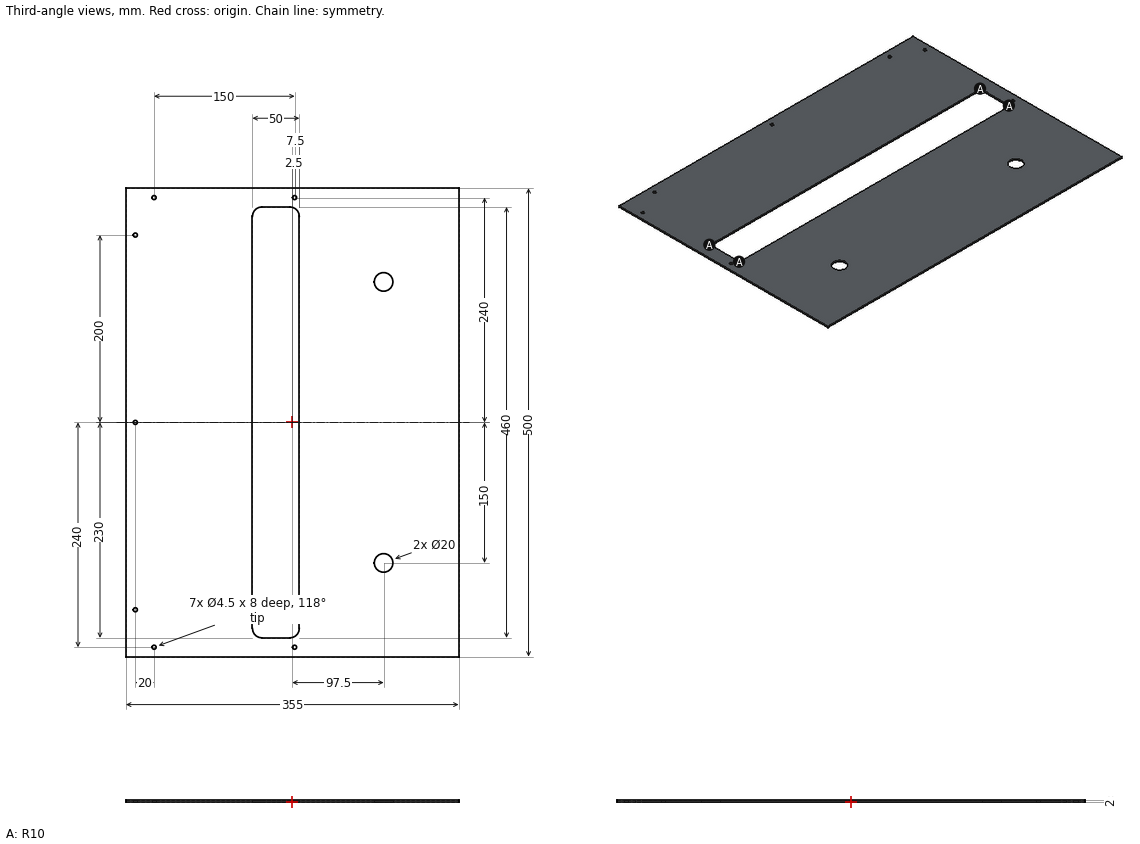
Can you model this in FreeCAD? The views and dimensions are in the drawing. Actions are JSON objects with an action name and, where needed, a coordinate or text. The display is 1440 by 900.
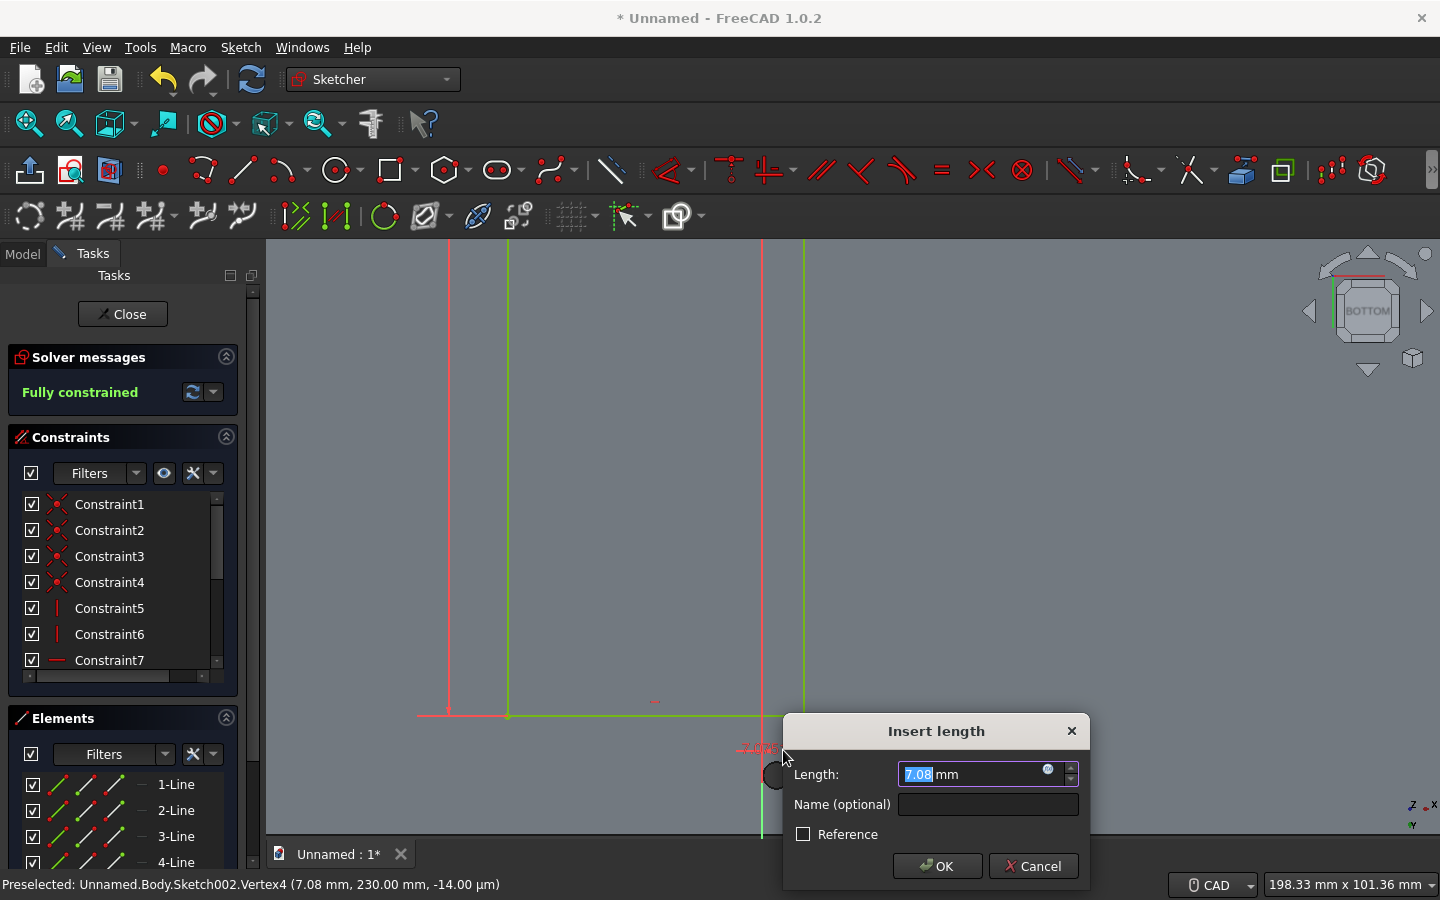
{"action": "type", "text": "7.5"}
{"action": "key", "text": "Return"}
{"action": "key", "text": "Escape"}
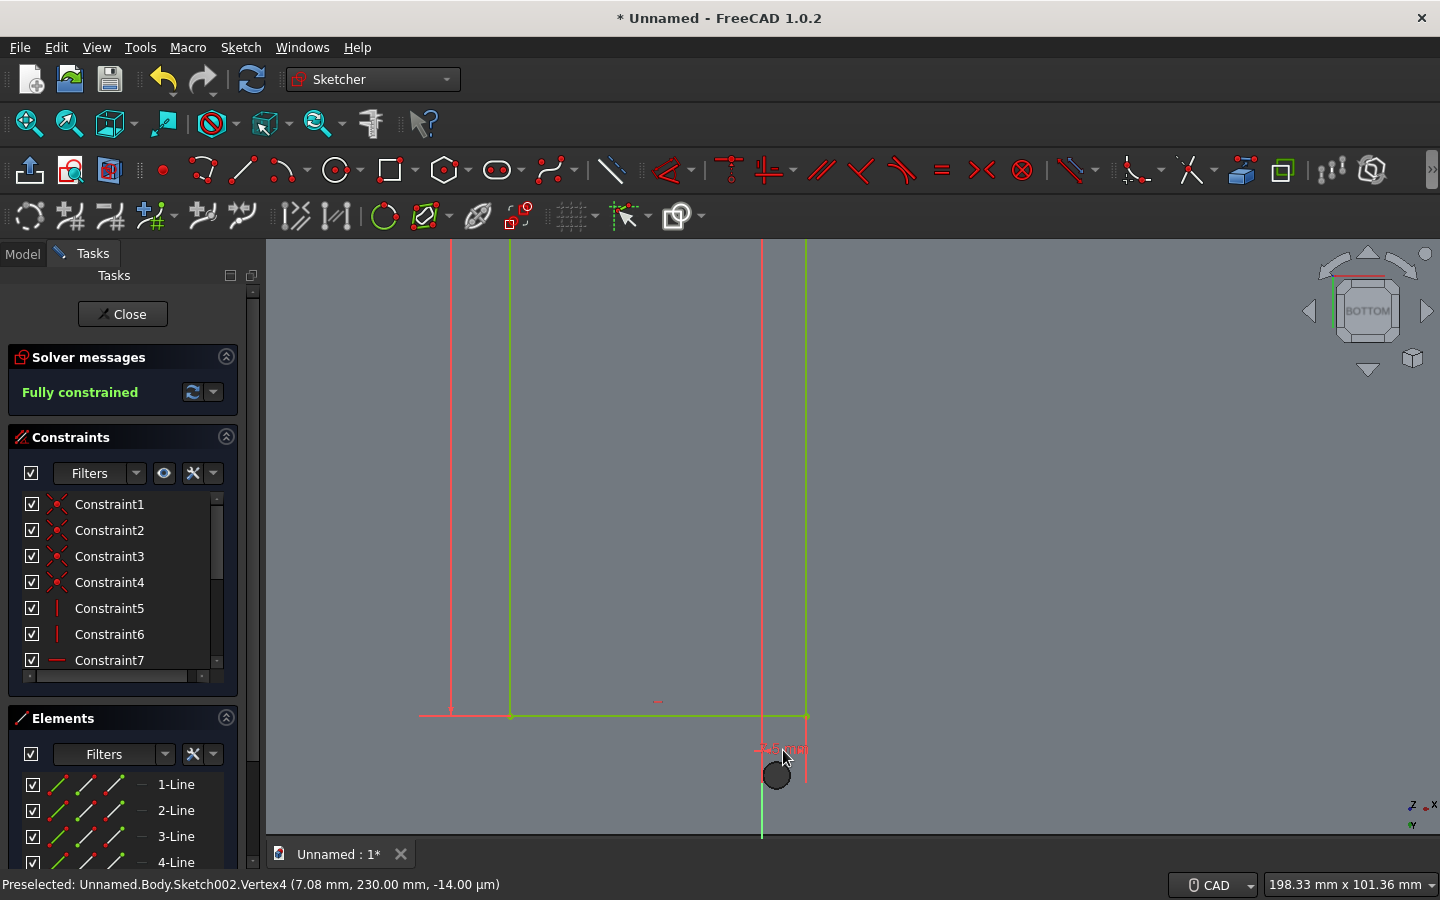
{"action": "left_click", "coordinate": [123, 314]}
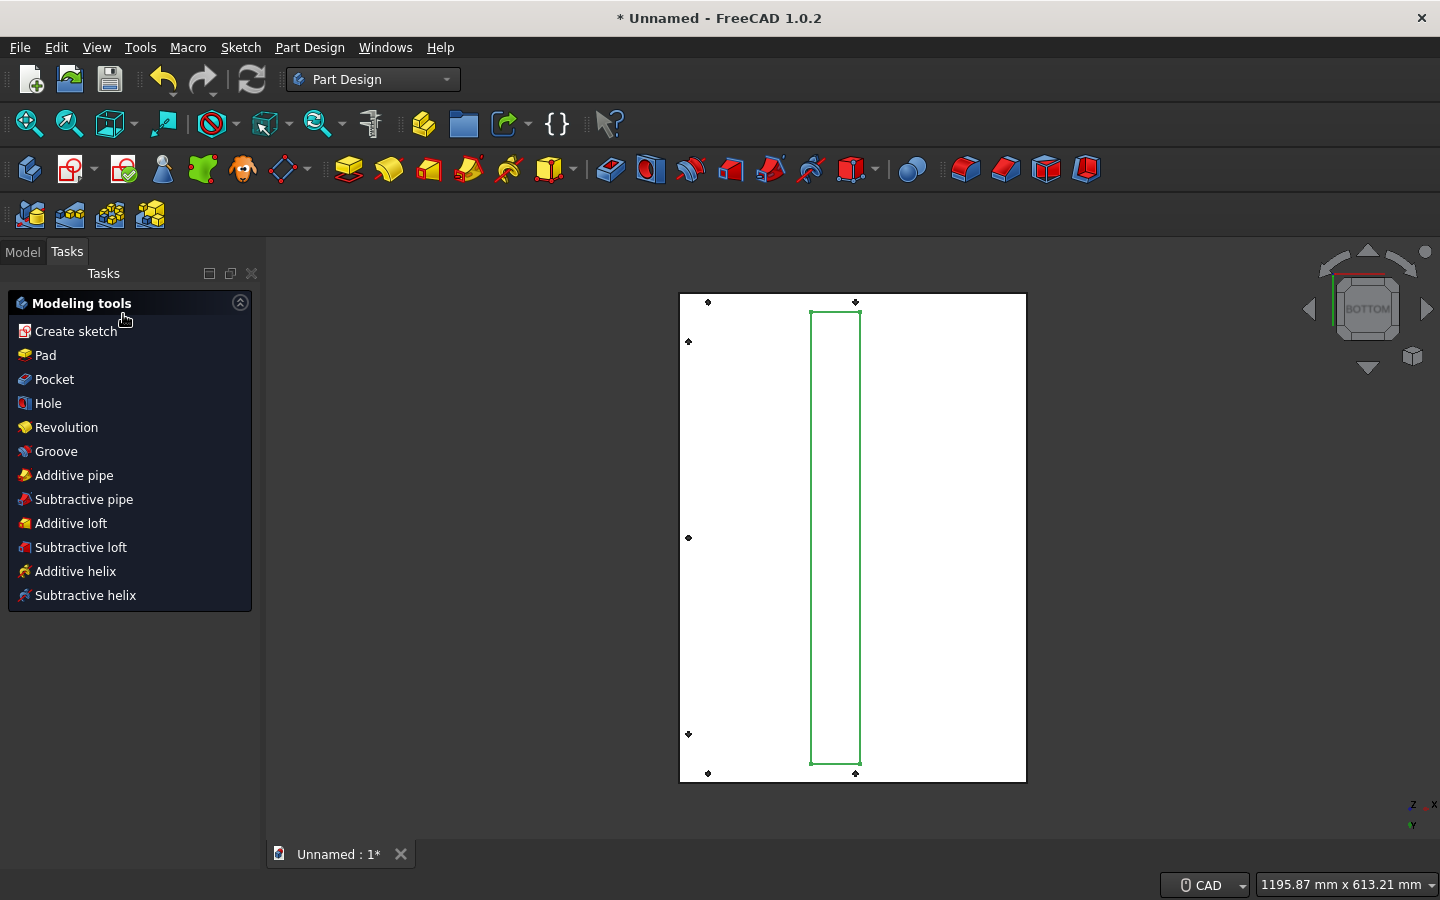
{"action": "left_click", "coordinate": [612, 170]}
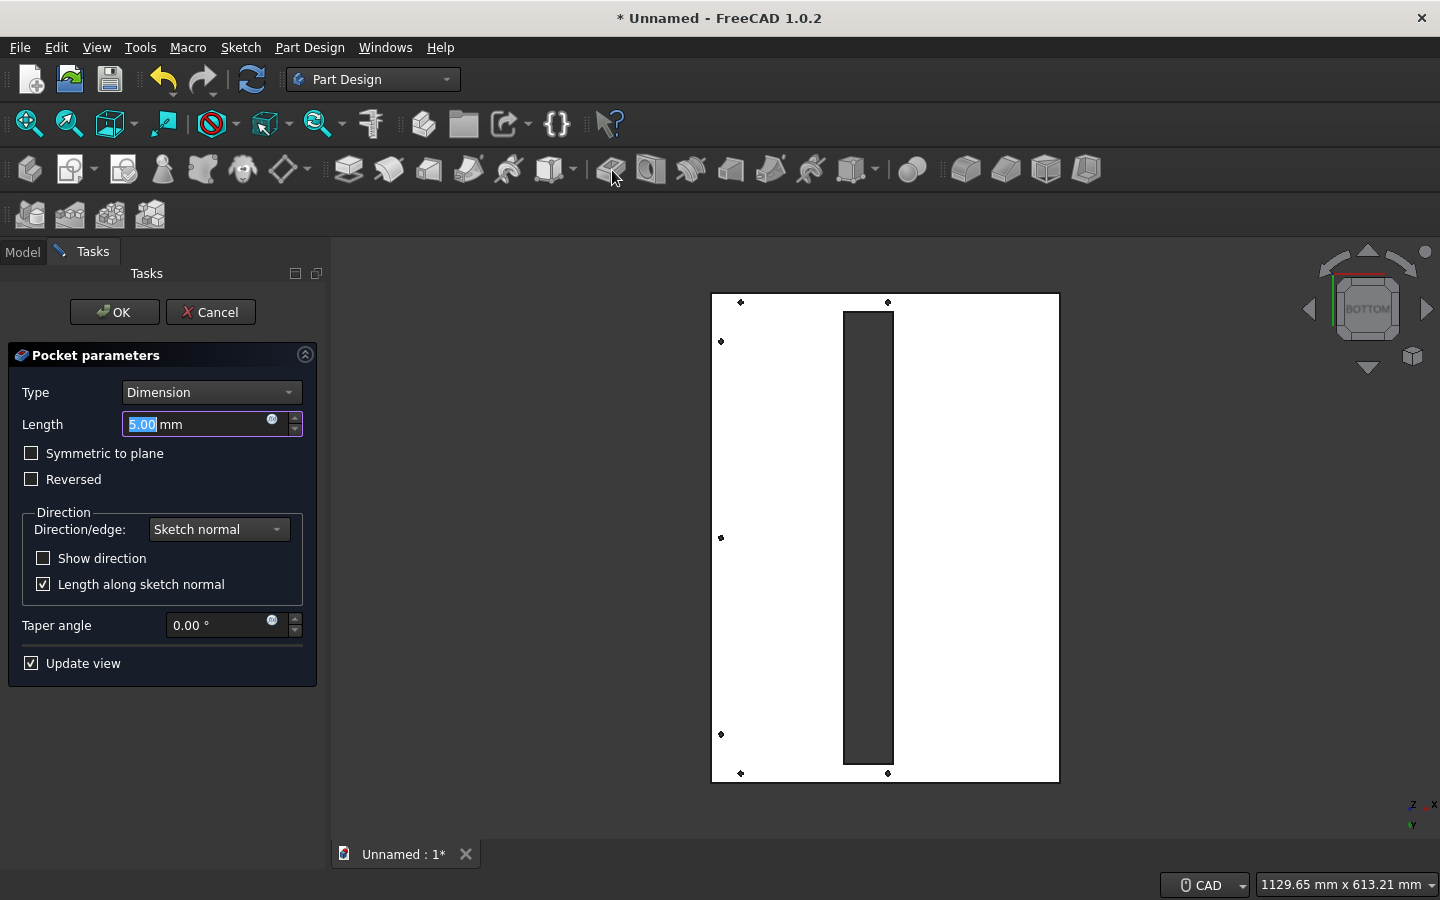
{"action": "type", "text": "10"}
{"action": "key", "text": "Tab"}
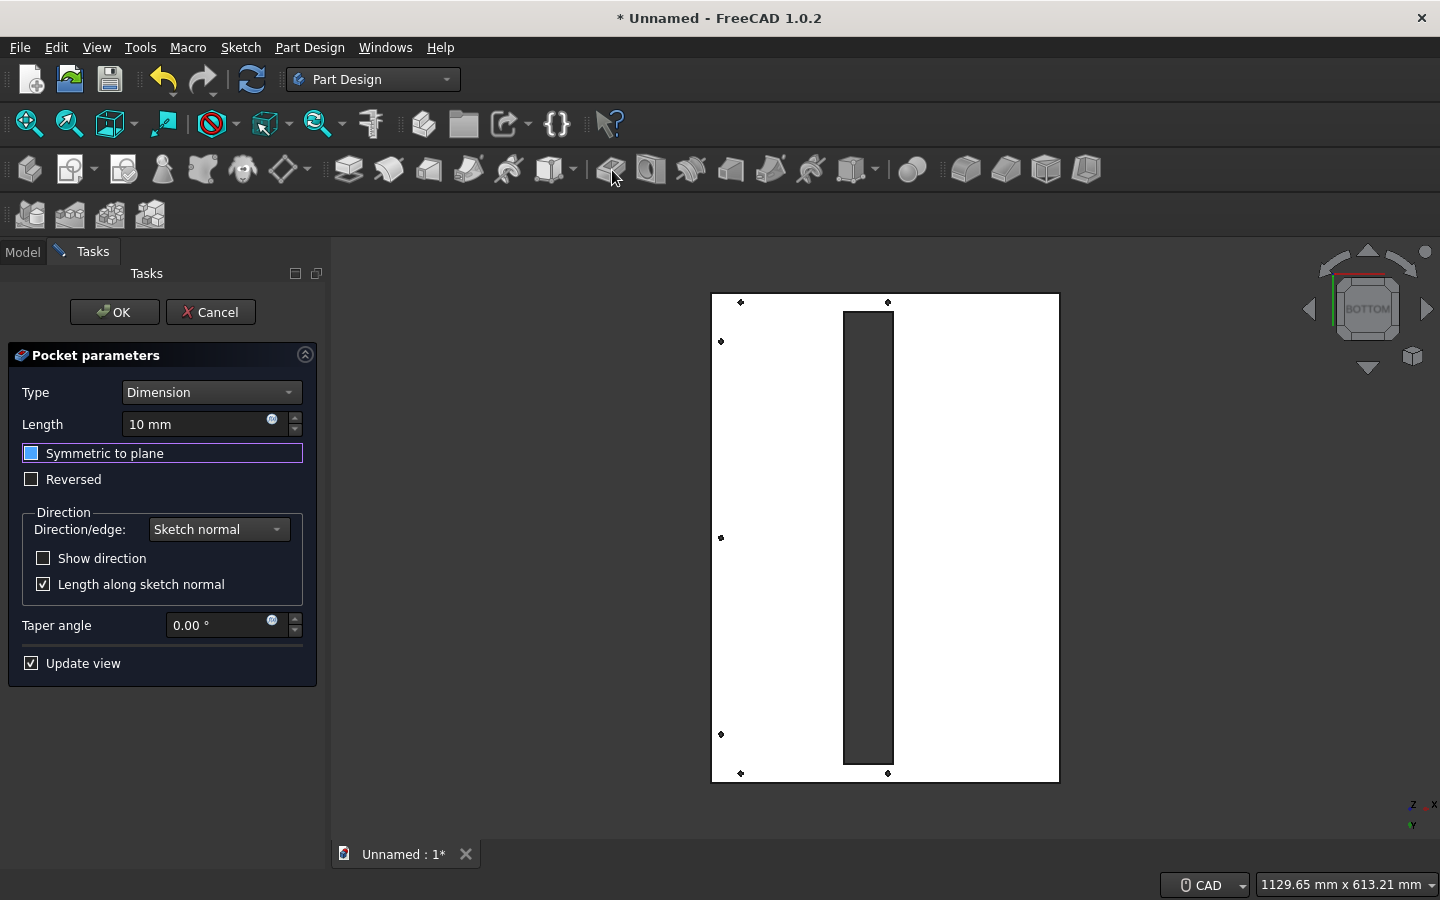
{"action": "left_click", "coordinate": [115, 312]}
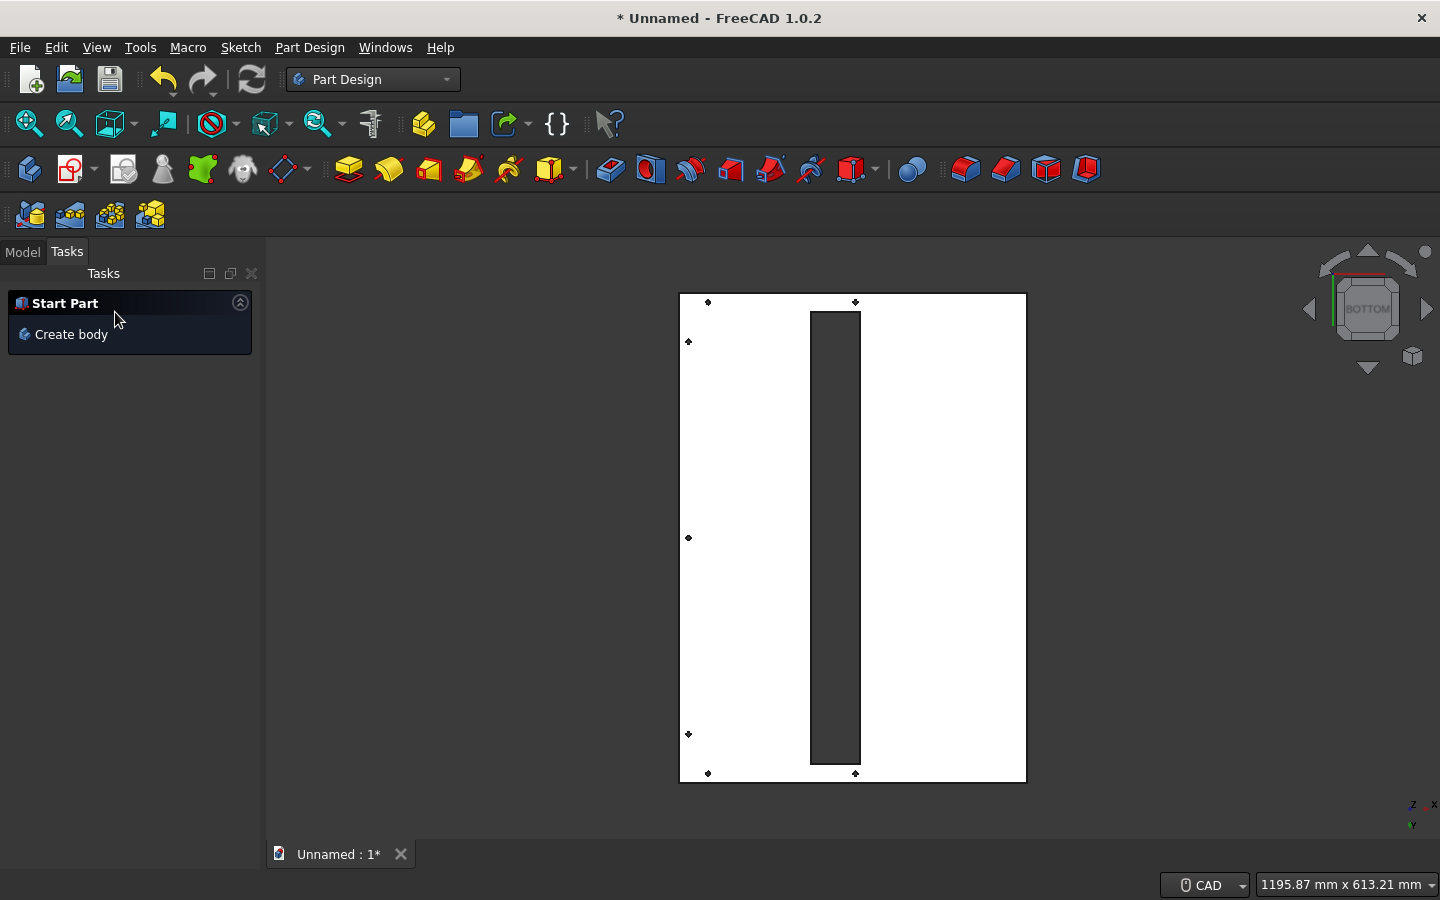
{"action": "scroll", "coordinate": [811, 763], "scroll_direction": "up", "scroll_amount": 15}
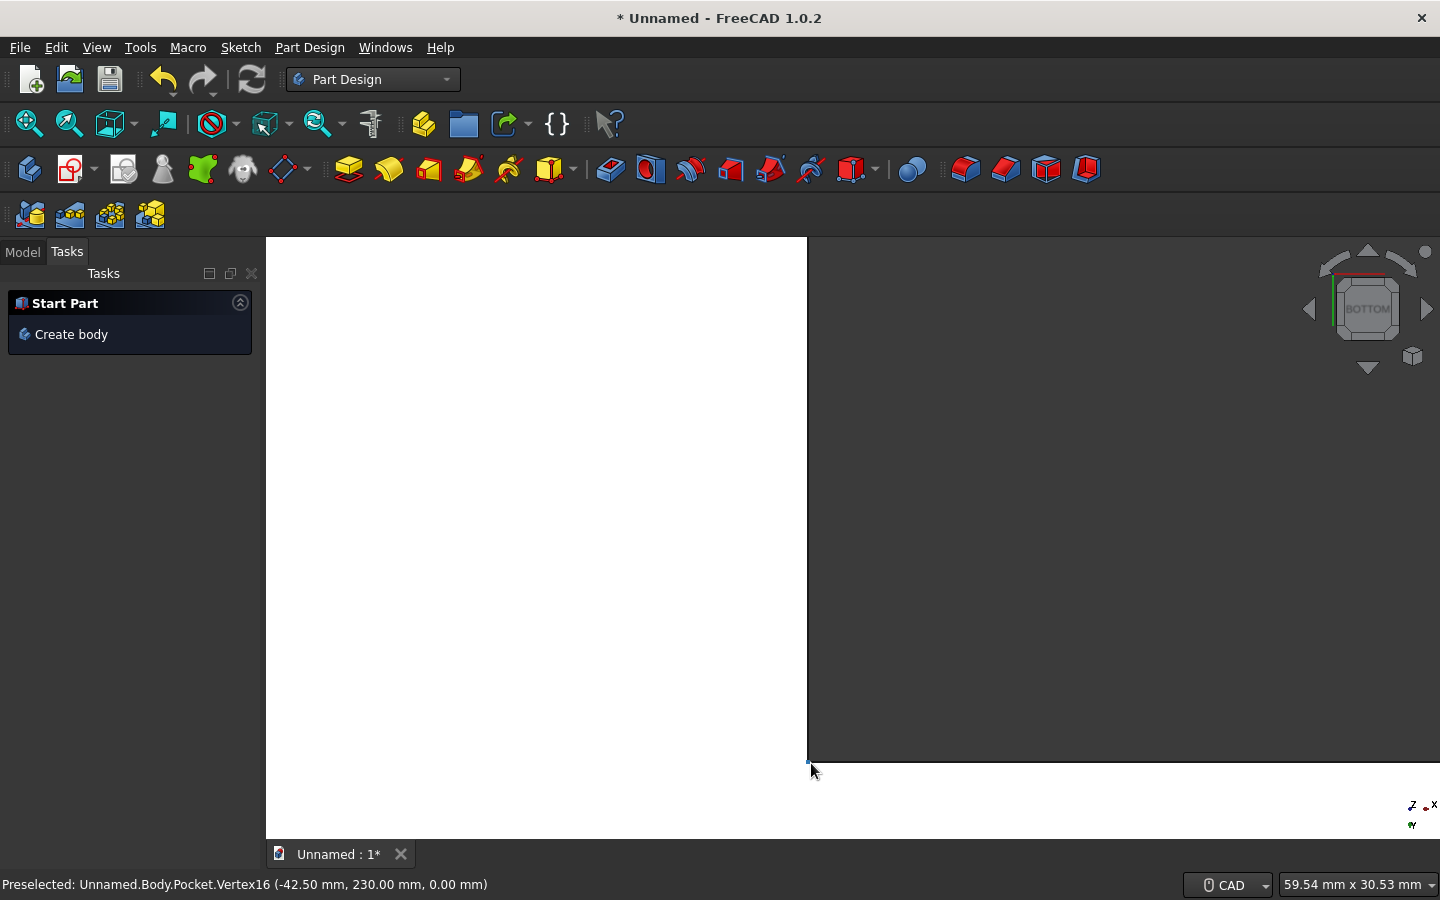
{"action": "left_click", "coordinate": [30, 124]}